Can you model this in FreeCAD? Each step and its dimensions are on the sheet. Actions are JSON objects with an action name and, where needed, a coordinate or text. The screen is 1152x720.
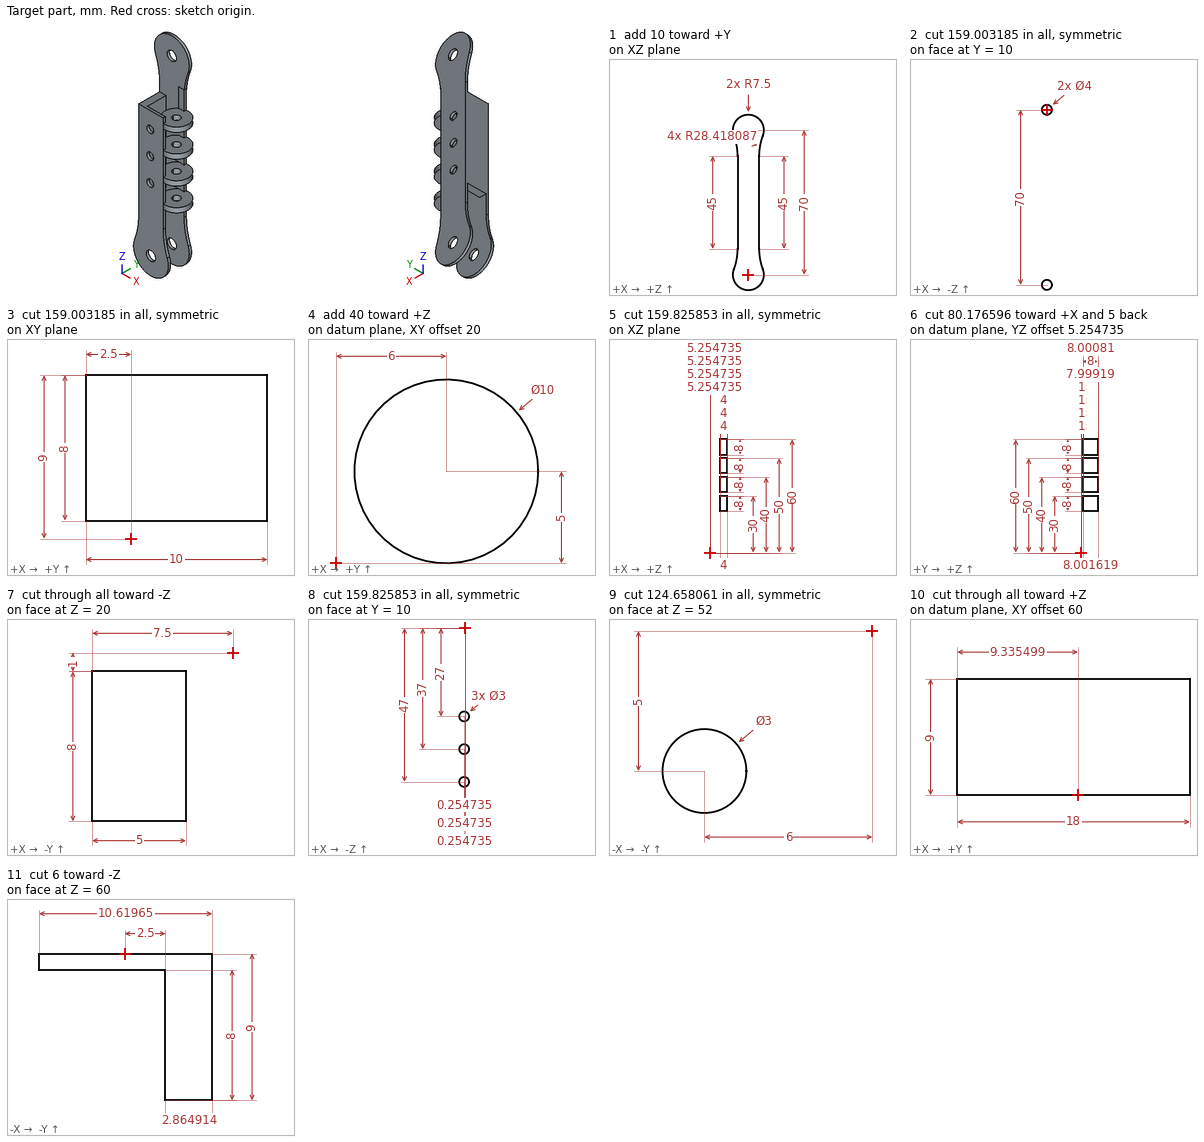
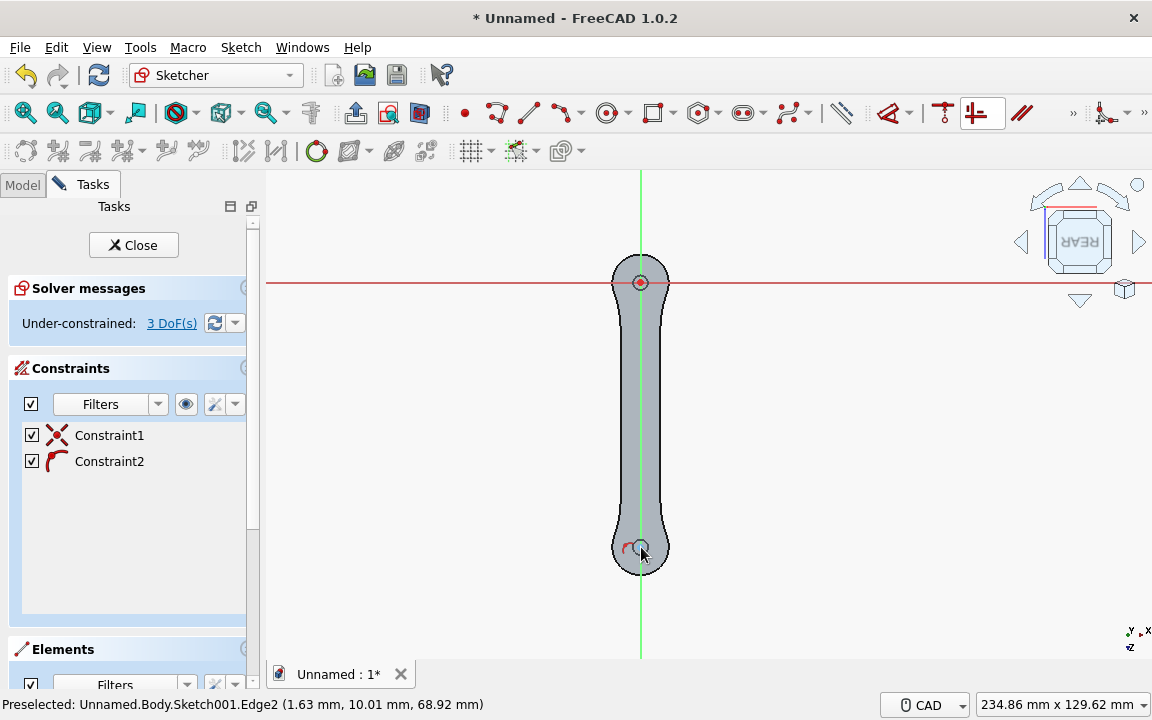
{"action": "scroll", "coordinate": [646, 278], "scroll_direction": "up", "scroll_amount": 5}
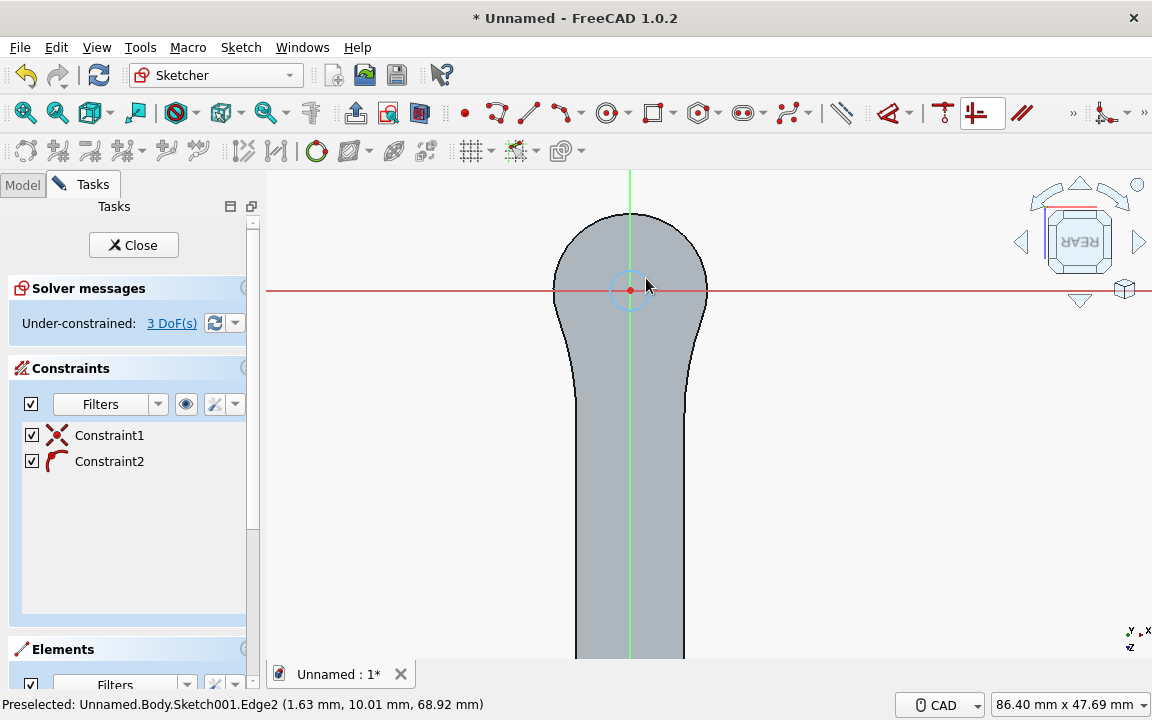
{"action": "left_click", "coordinate": [644, 277]}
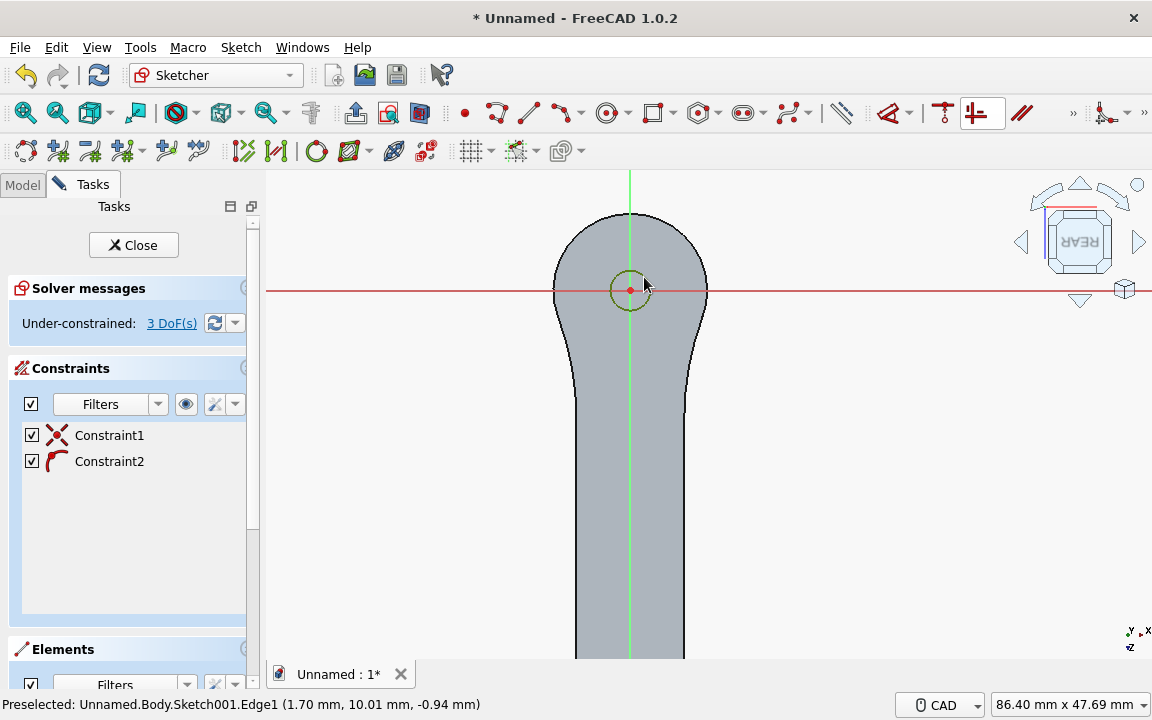
{"action": "scroll", "coordinate": [646, 278], "scroll_direction": "down", "scroll_amount": 5}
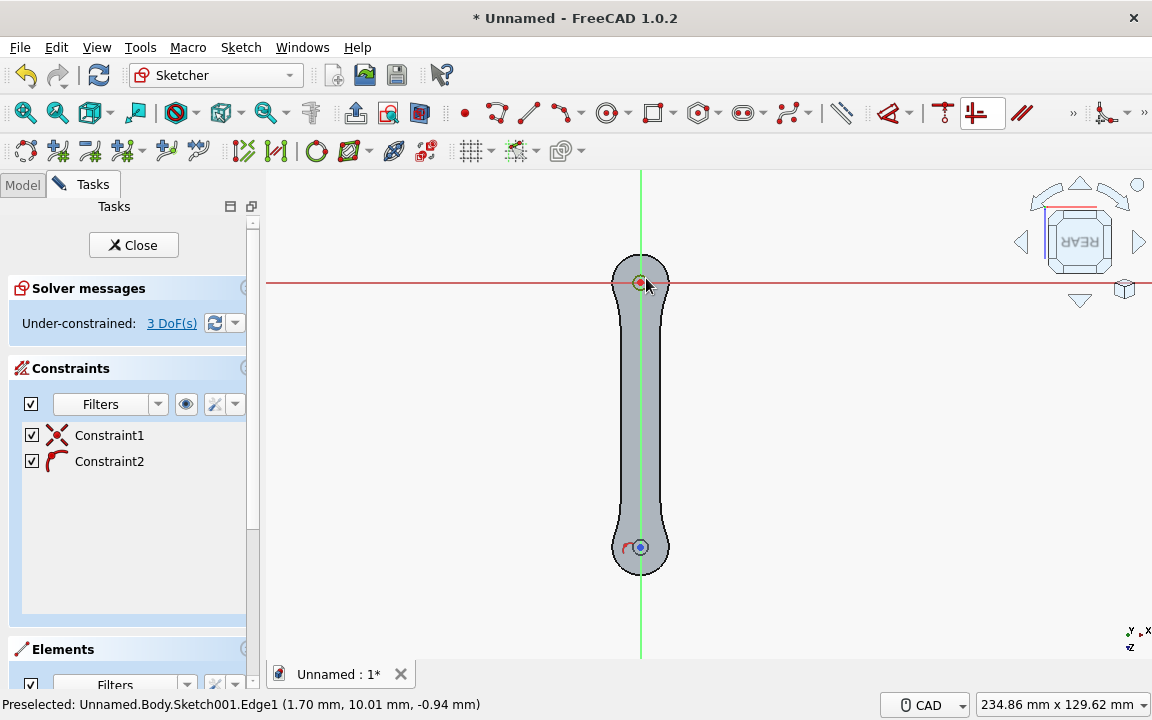
{"action": "scroll", "coordinate": [646, 542], "scroll_direction": "up", "scroll_amount": 5}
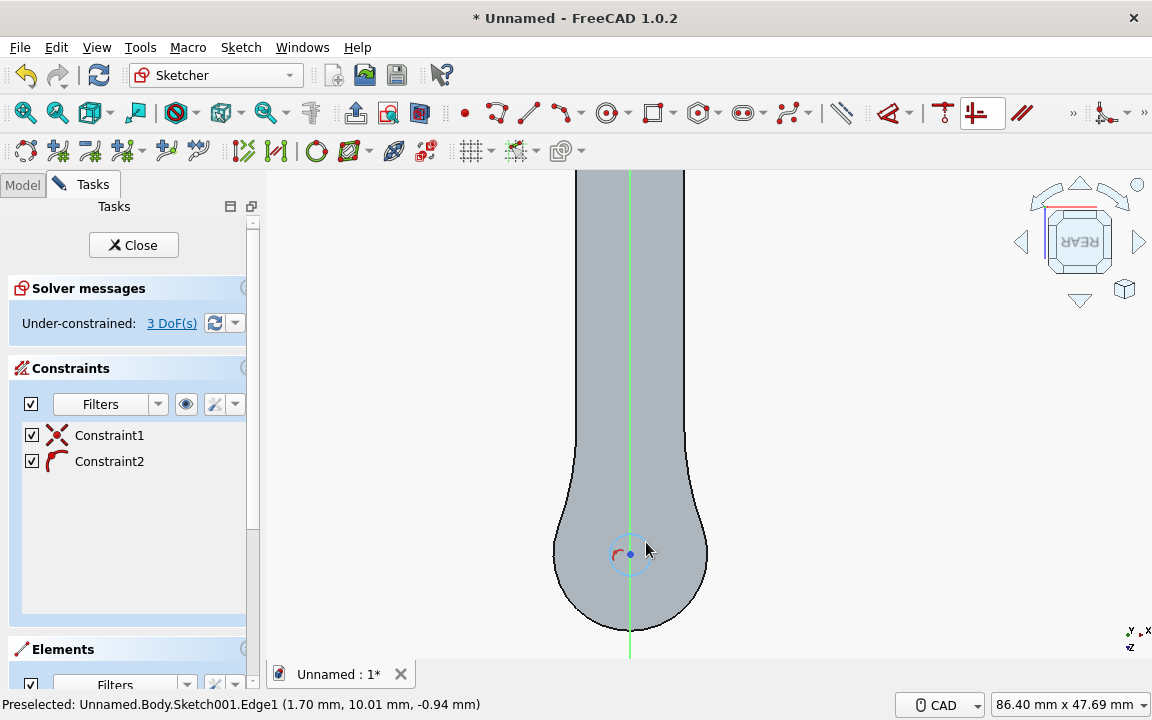
{"action": "left_click", "coordinate": [645, 540]}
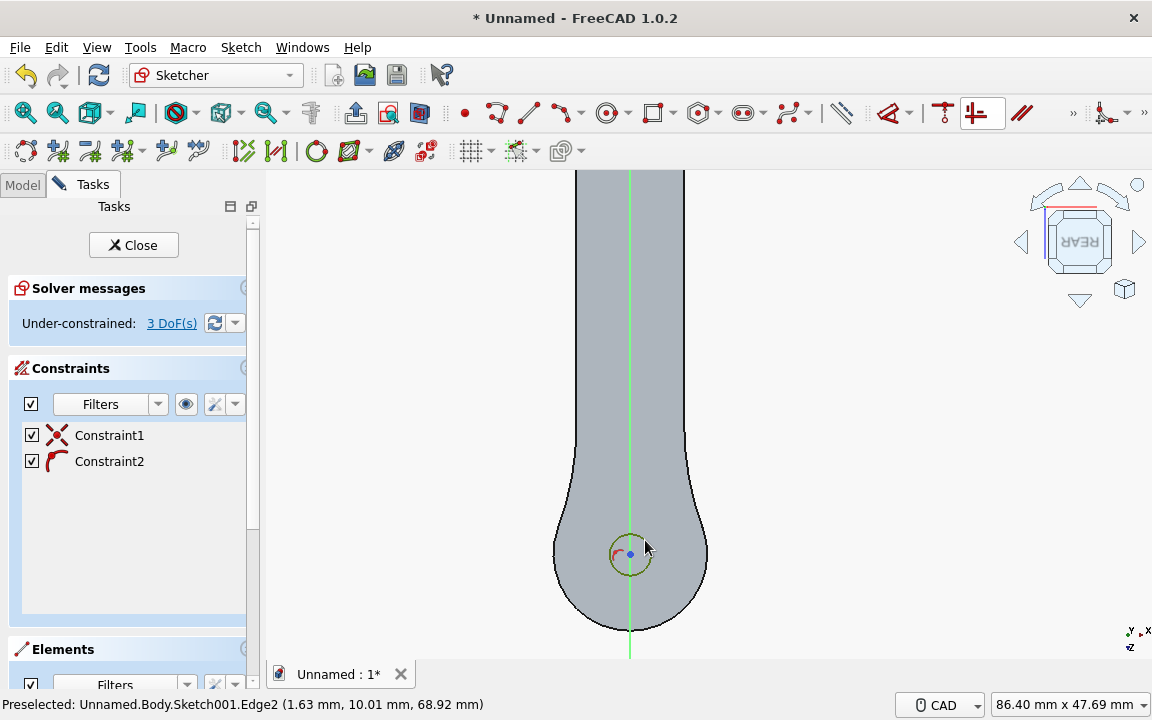
{"action": "key", "text": "e"}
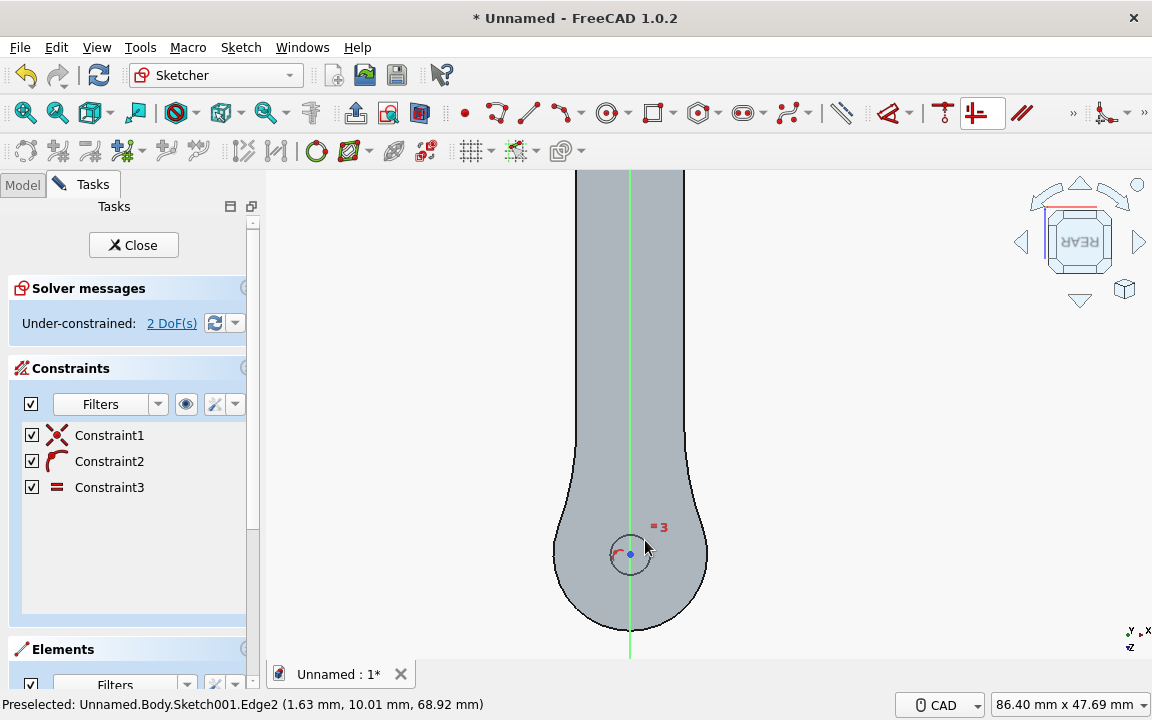
{"action": "left_click", "coordinate": [888, 114]}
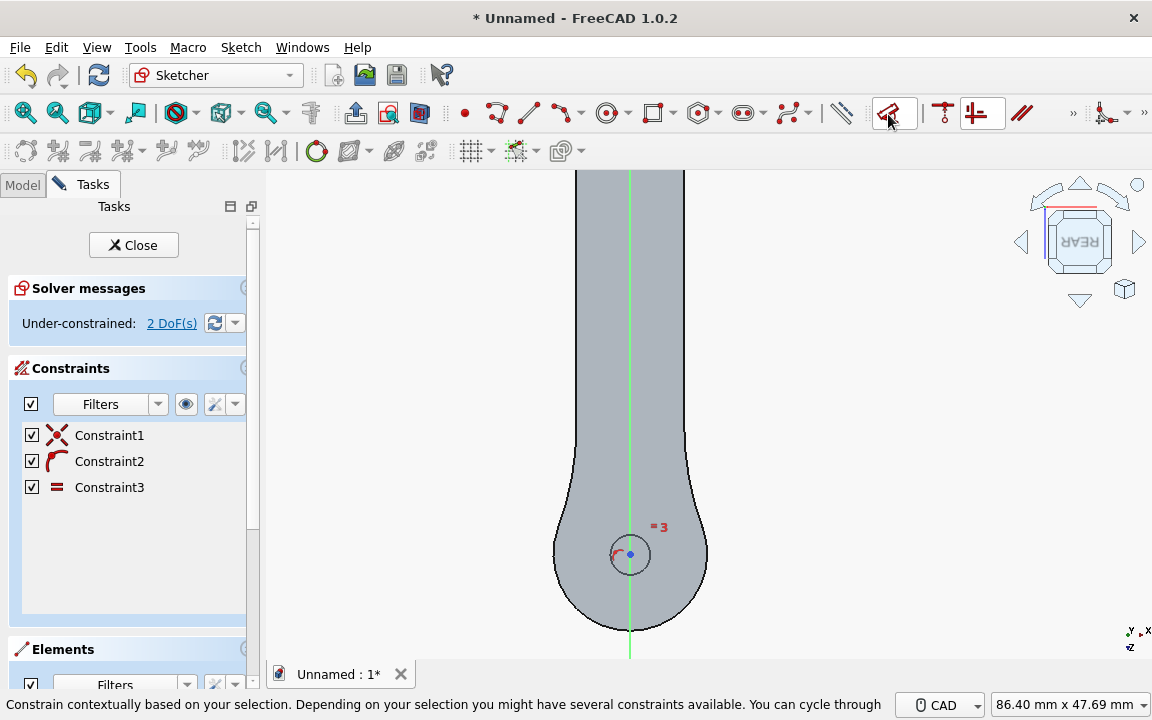
{"action": "scroll", "coordinate": [646, 542], "scroll_direction": "down", "scroll_amount": 5}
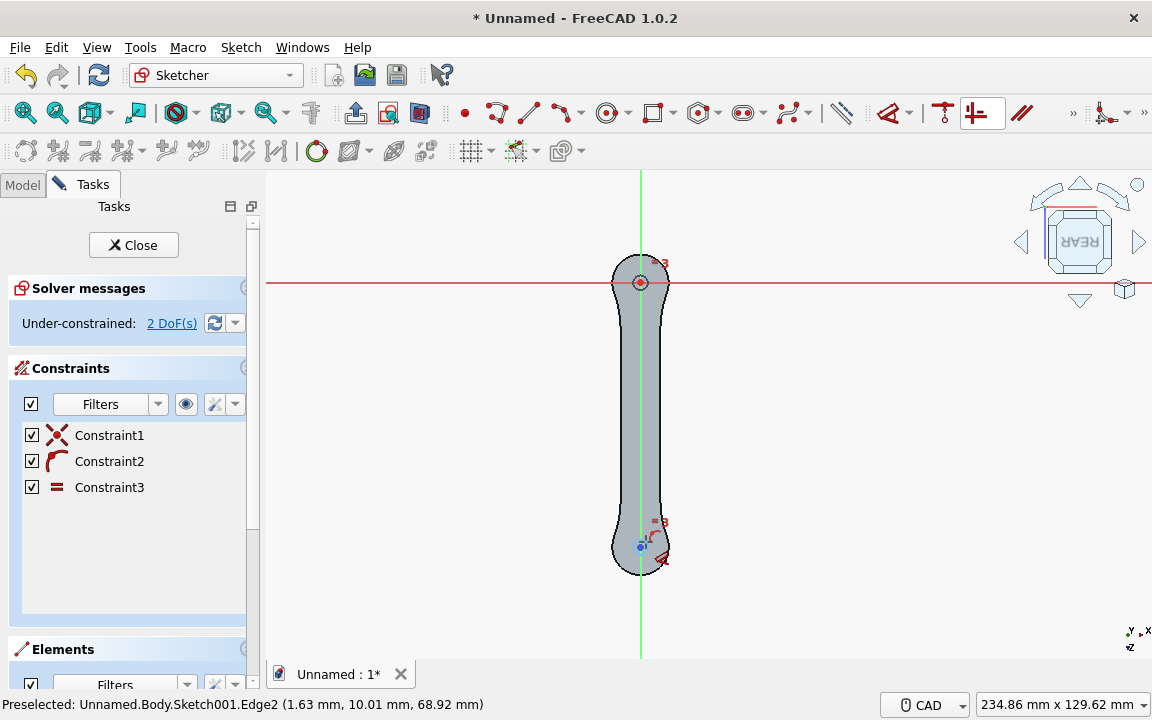
{"action": "scroll", "coordinate": [646, 278], "scroll_direction": "up", "scroll_amount": 5}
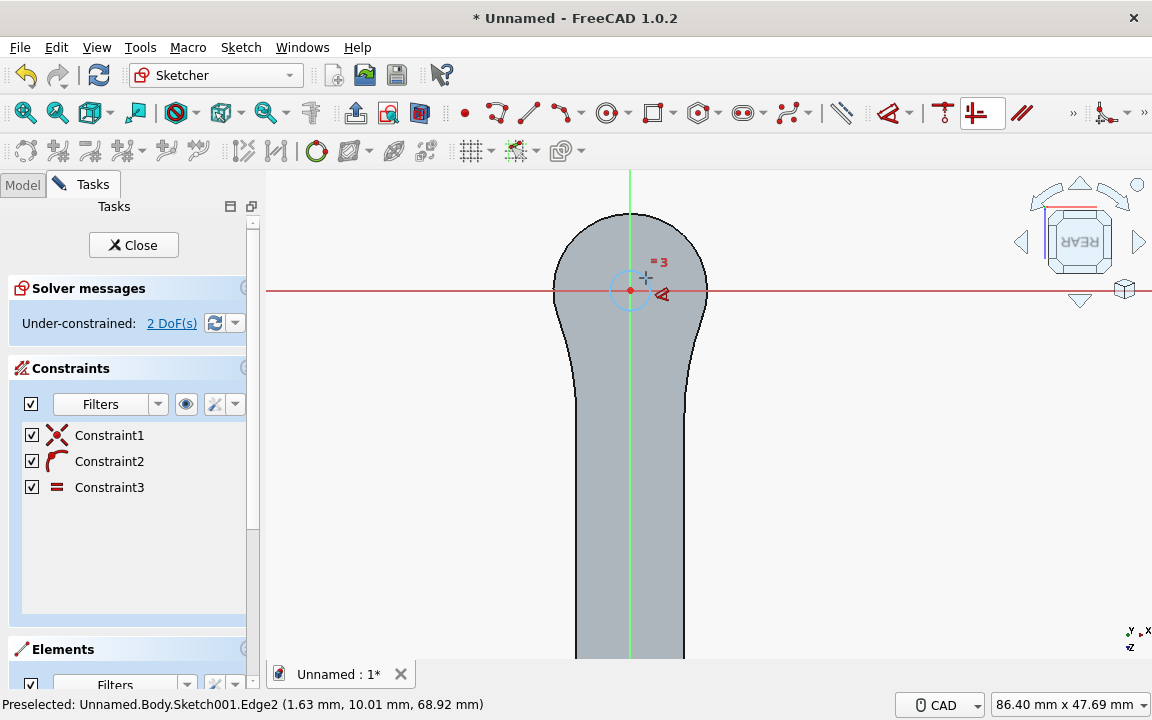
{"action": "left_click", "coordinate": [644, 277]}
{"action": "left_click", "coordinate": [667, 254]}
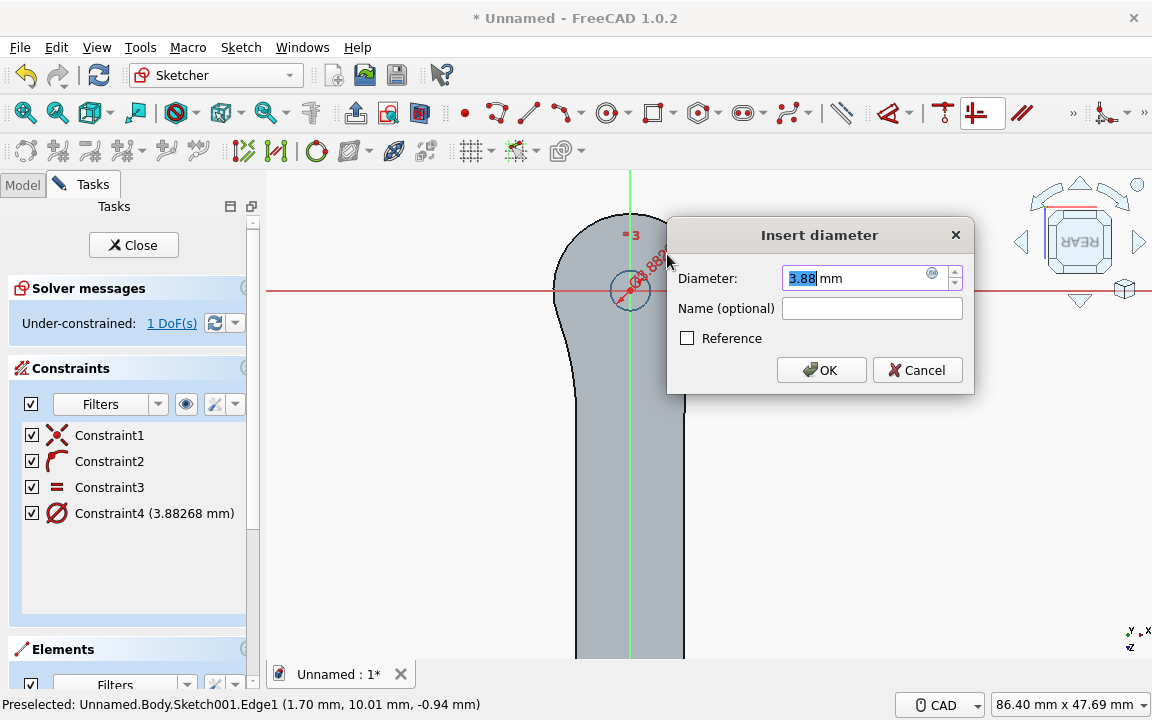
{"action": "type", "text": "4"}
{"action": "key", "text": "Return"}